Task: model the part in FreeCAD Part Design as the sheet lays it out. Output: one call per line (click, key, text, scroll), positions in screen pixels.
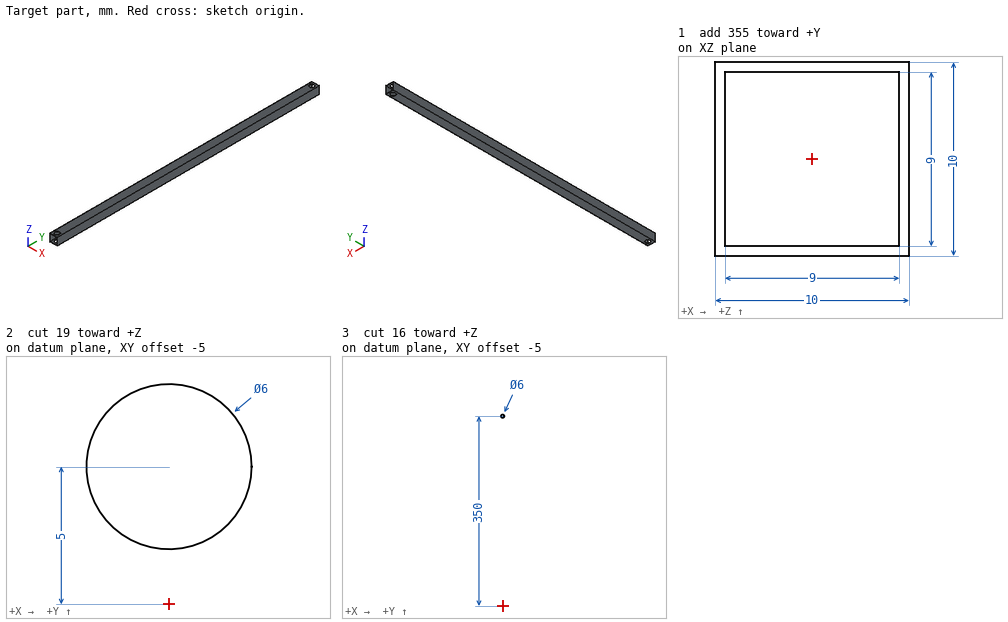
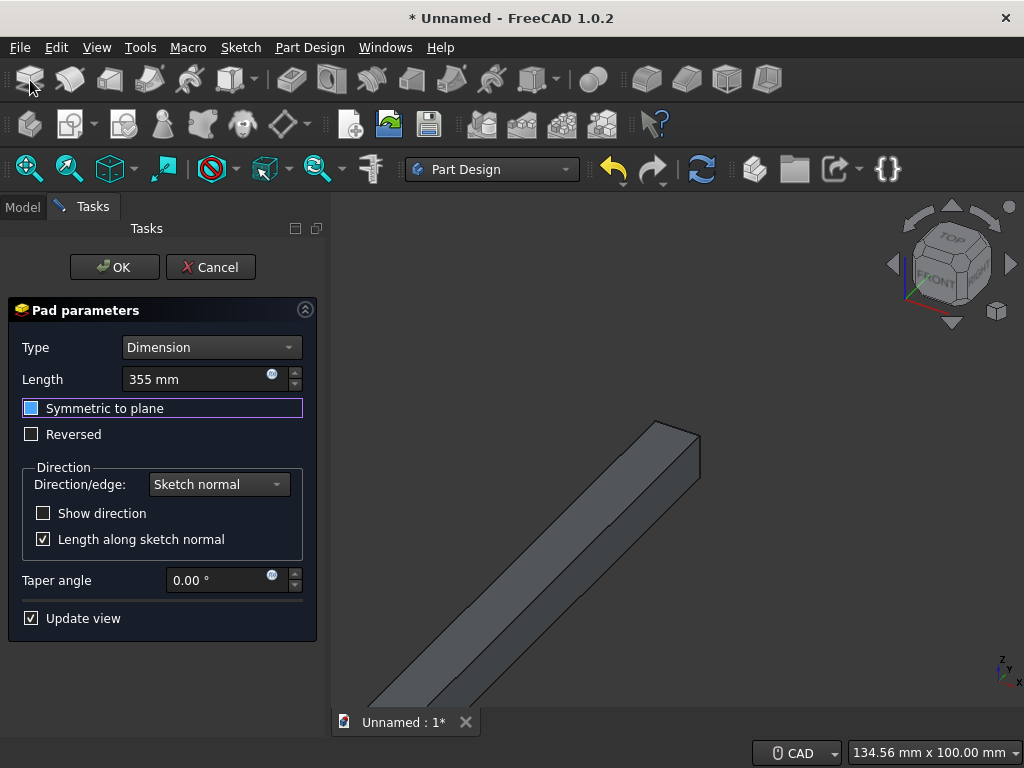
click(30, 434)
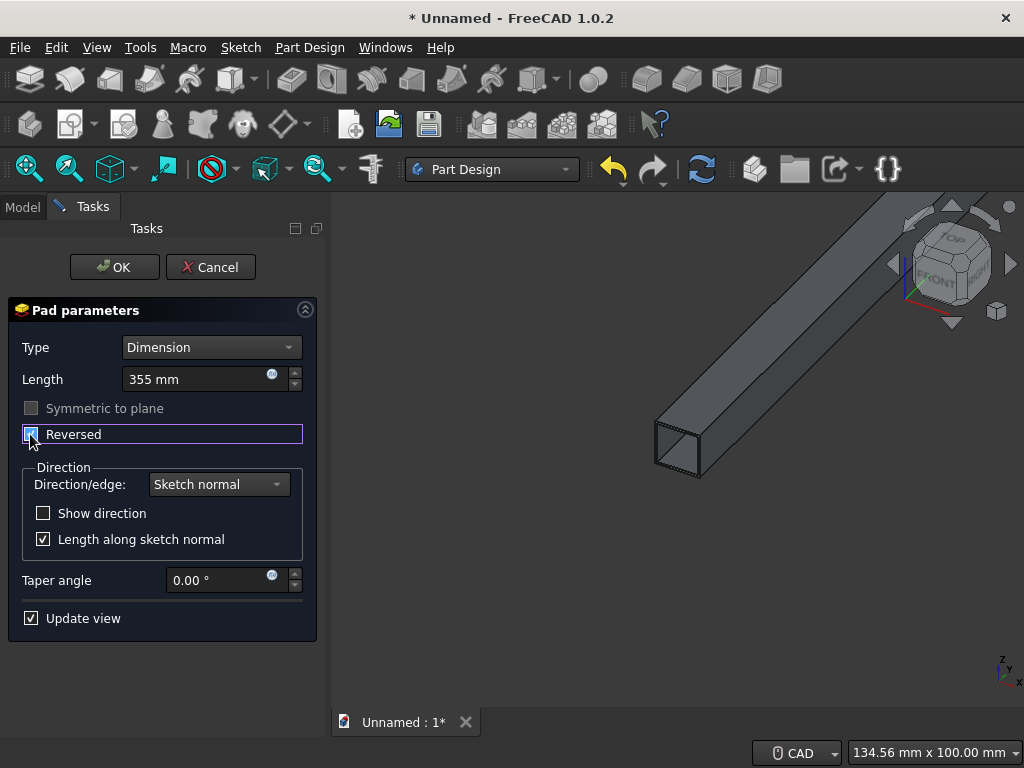
click(115, 267)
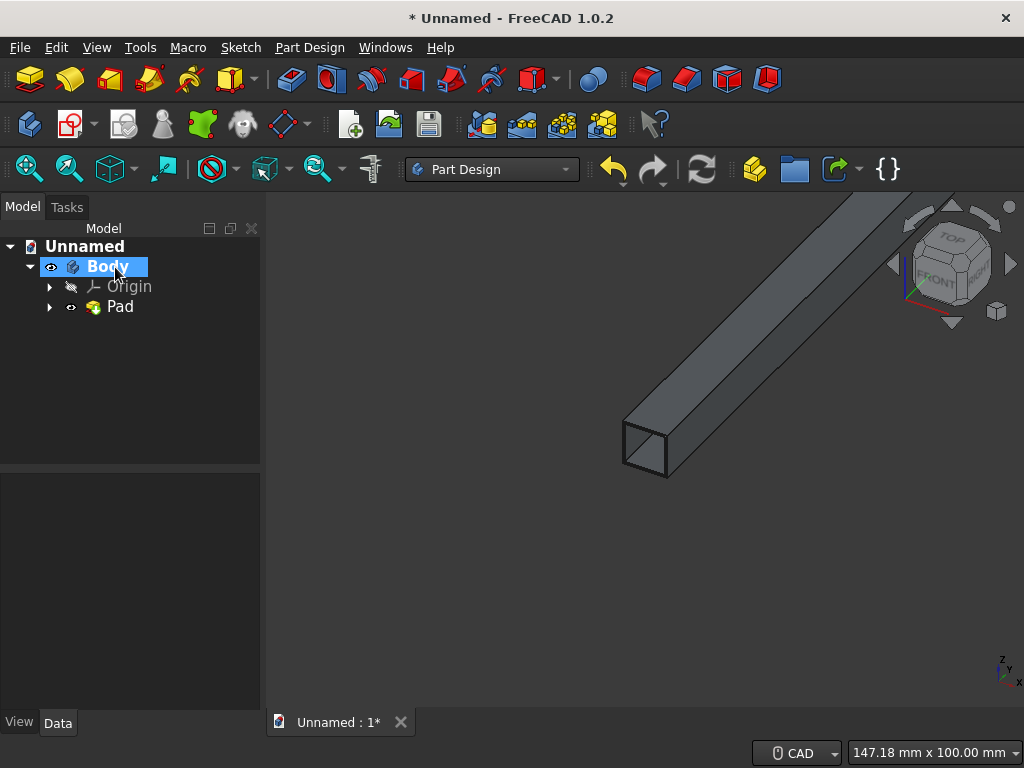
click(30, 170)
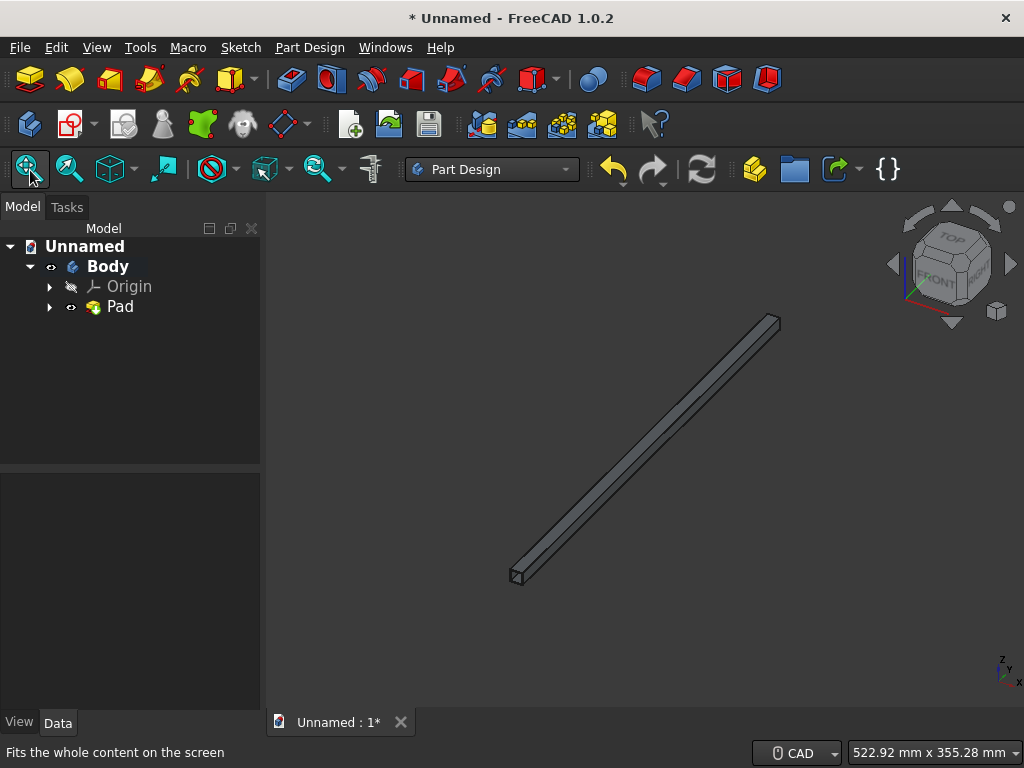
key(5)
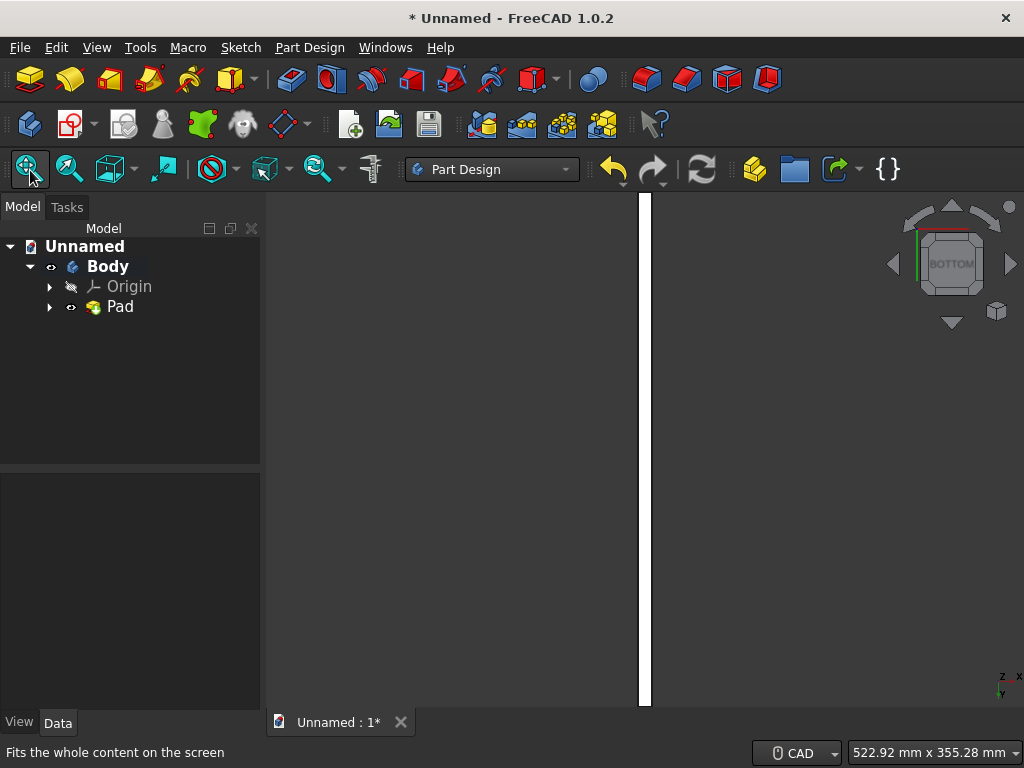
click(30, 170)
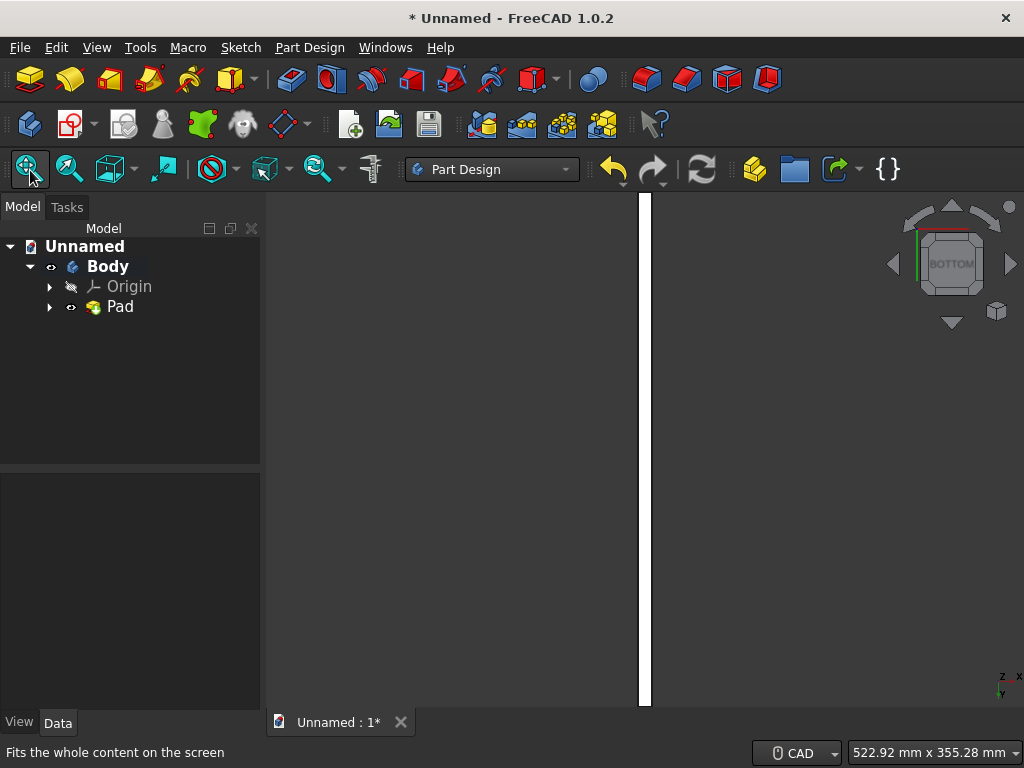
key(1)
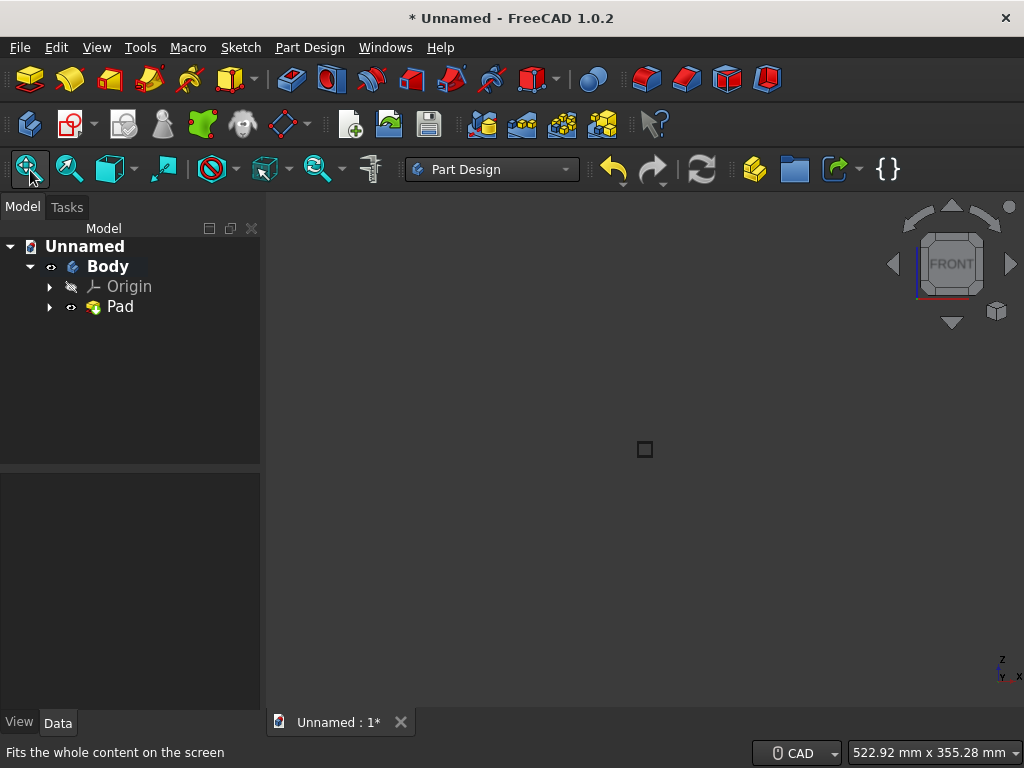
click(30, 170)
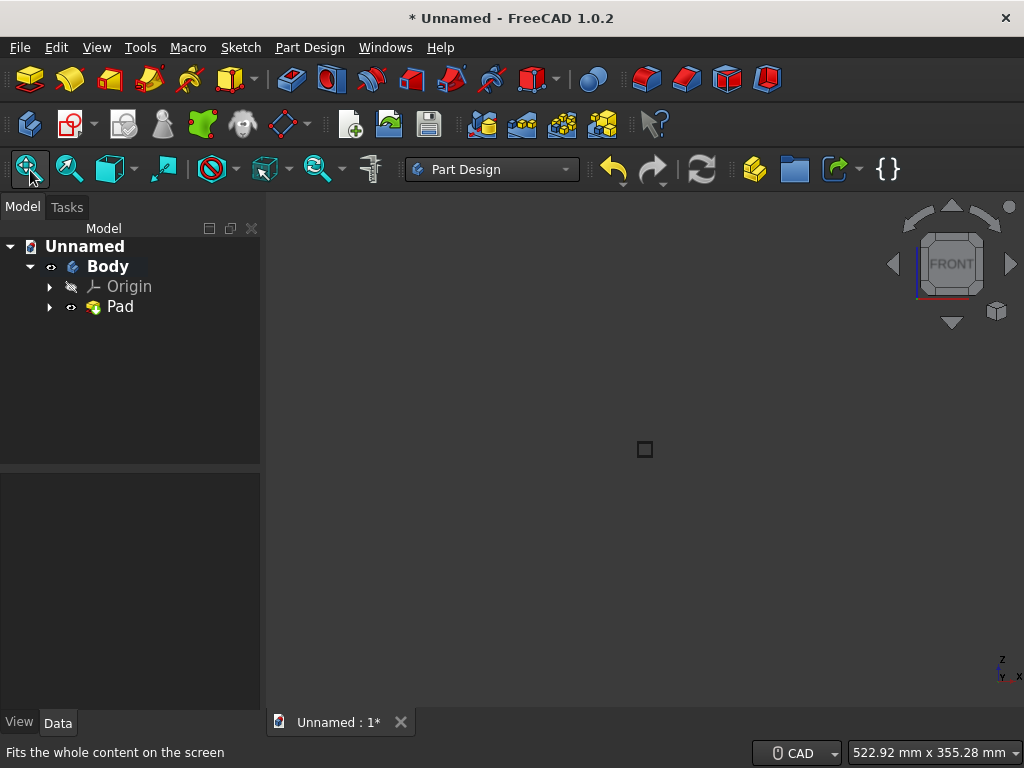
key(3)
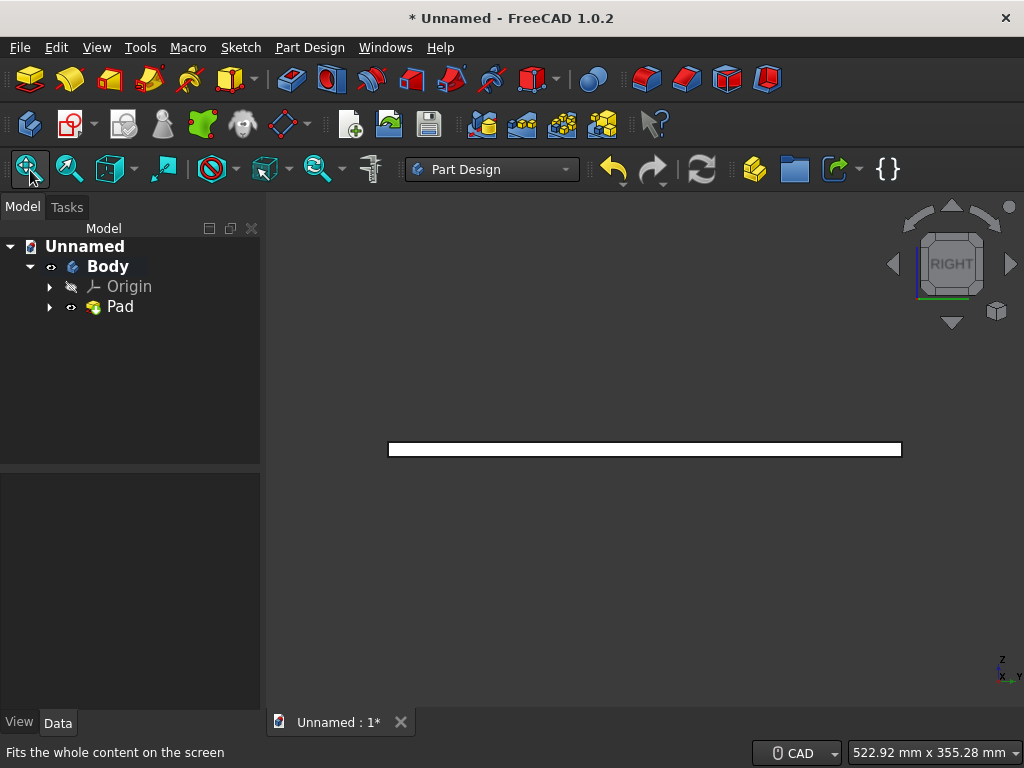
click(50, 287)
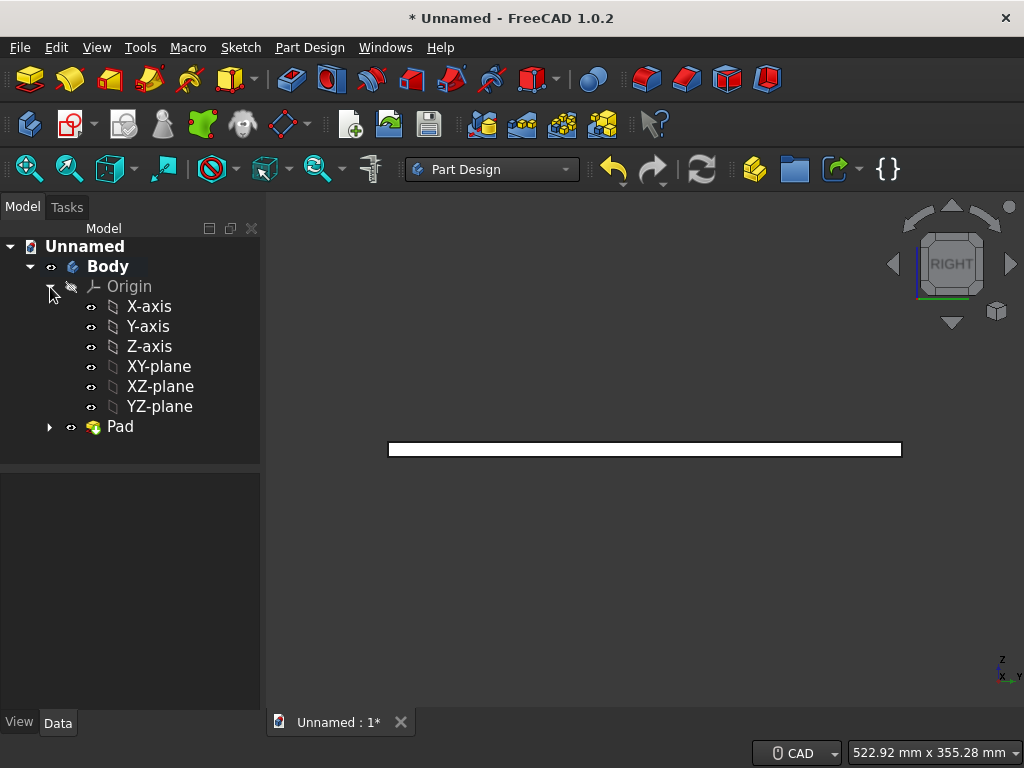
click(136, 367)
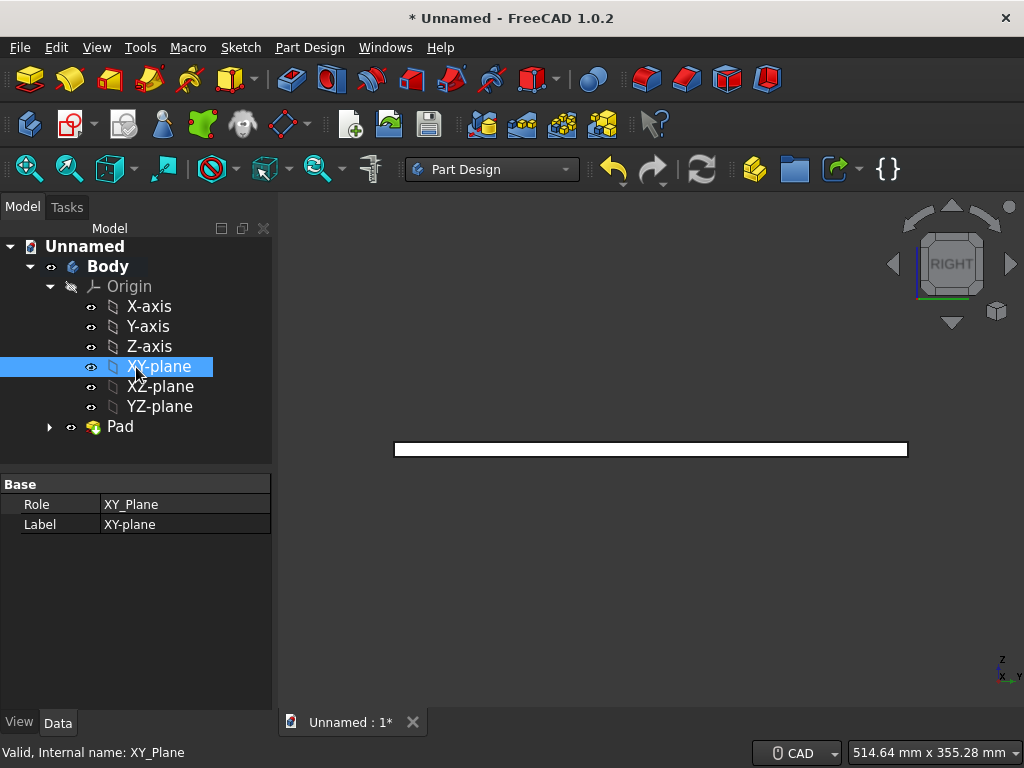
click(284, 124)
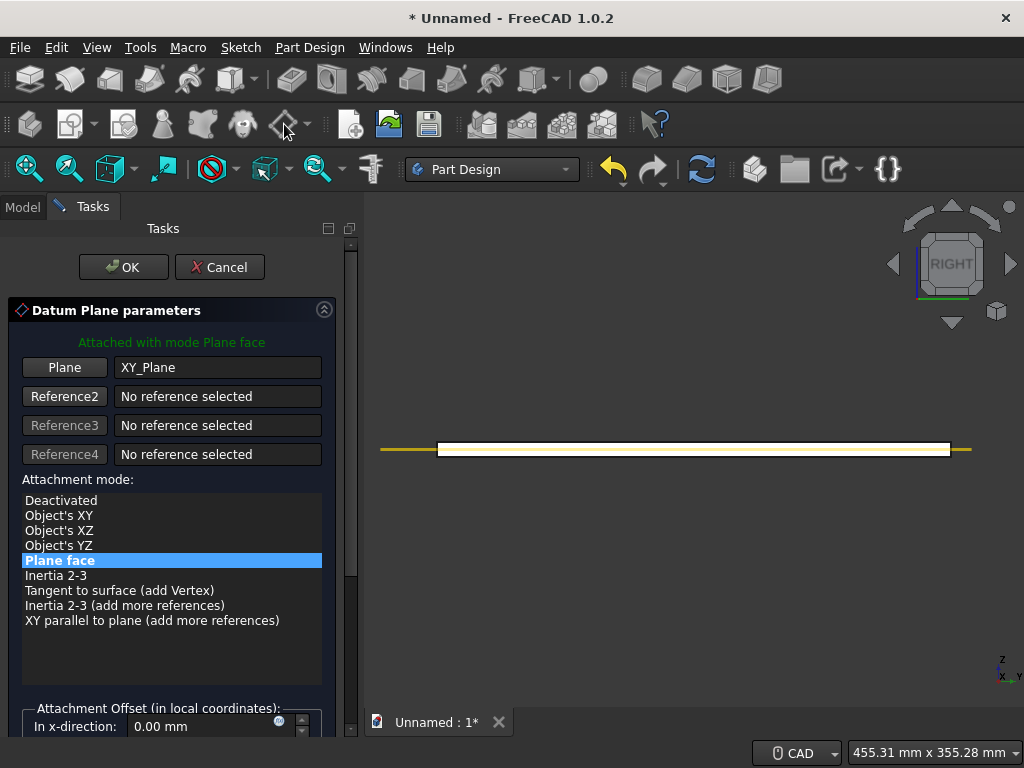
scroll(351, 487, down, 3)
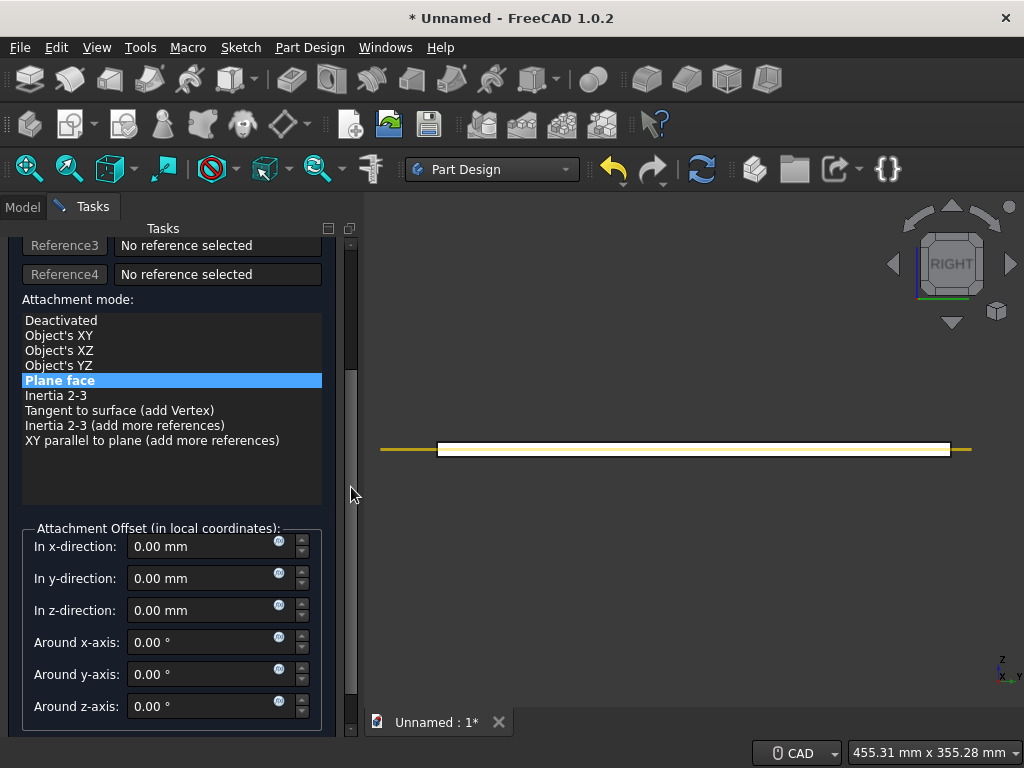
triple_click(210, 610)